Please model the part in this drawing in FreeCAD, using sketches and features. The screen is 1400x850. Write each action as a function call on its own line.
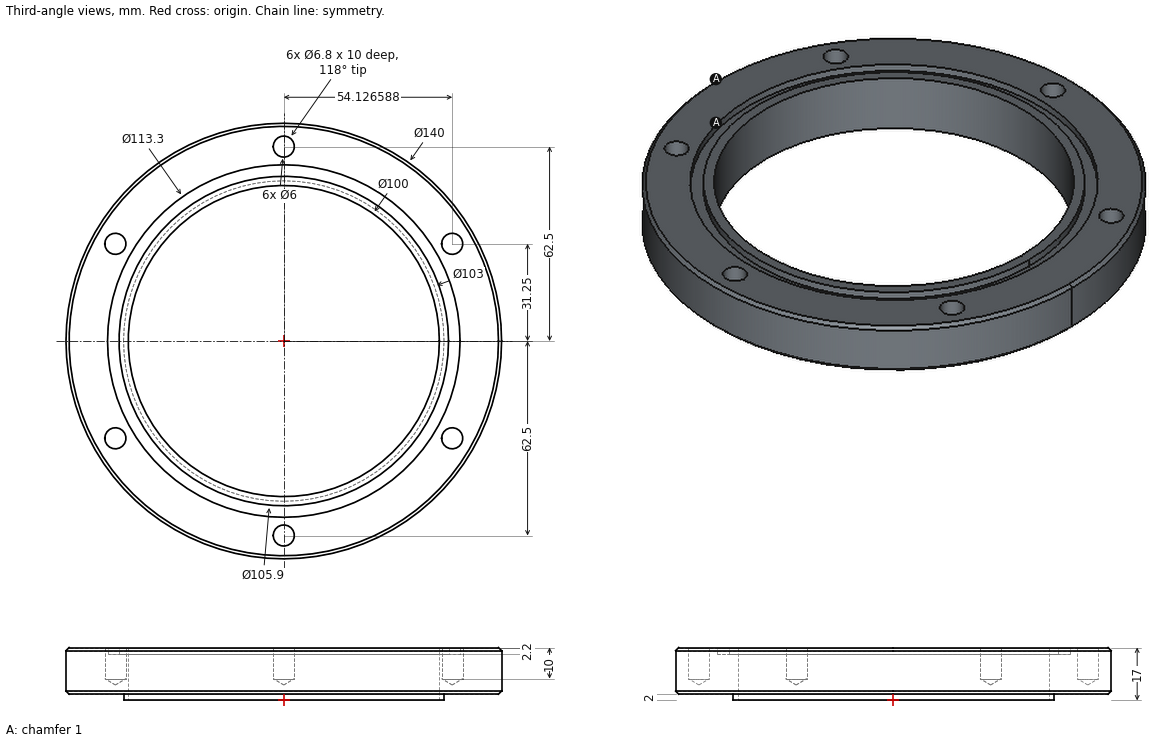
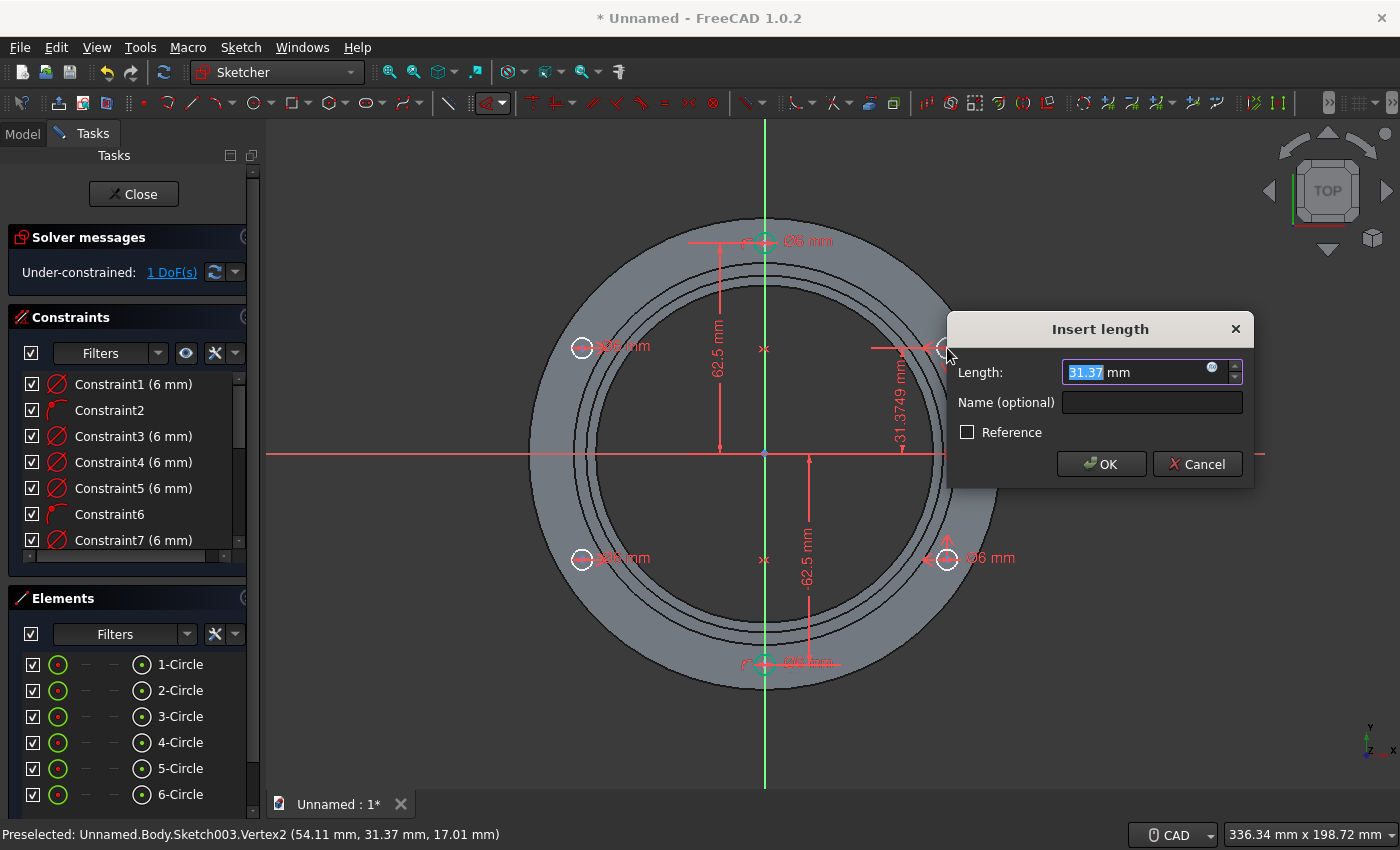
text(31.25)
key(Return)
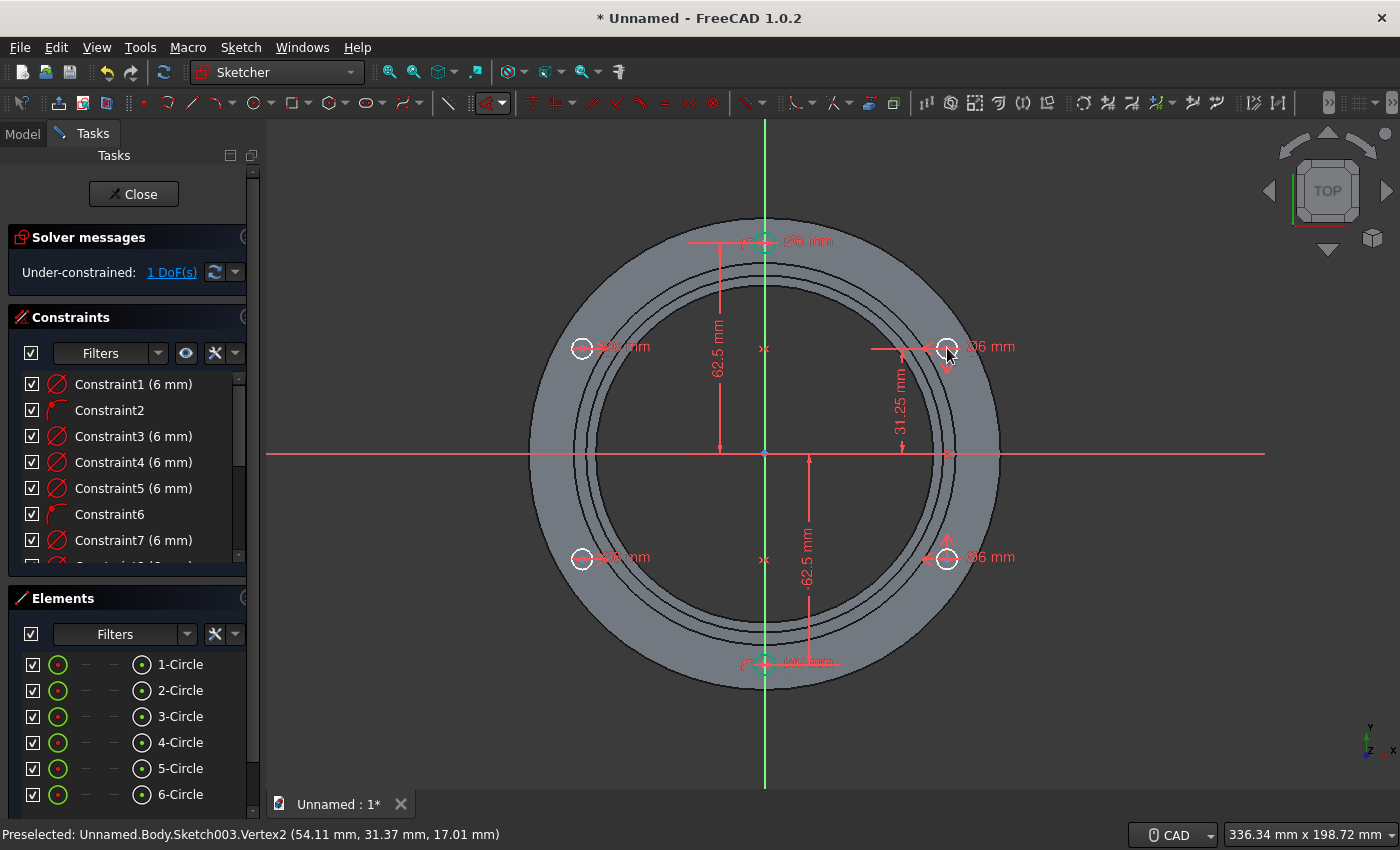
click(947, 349)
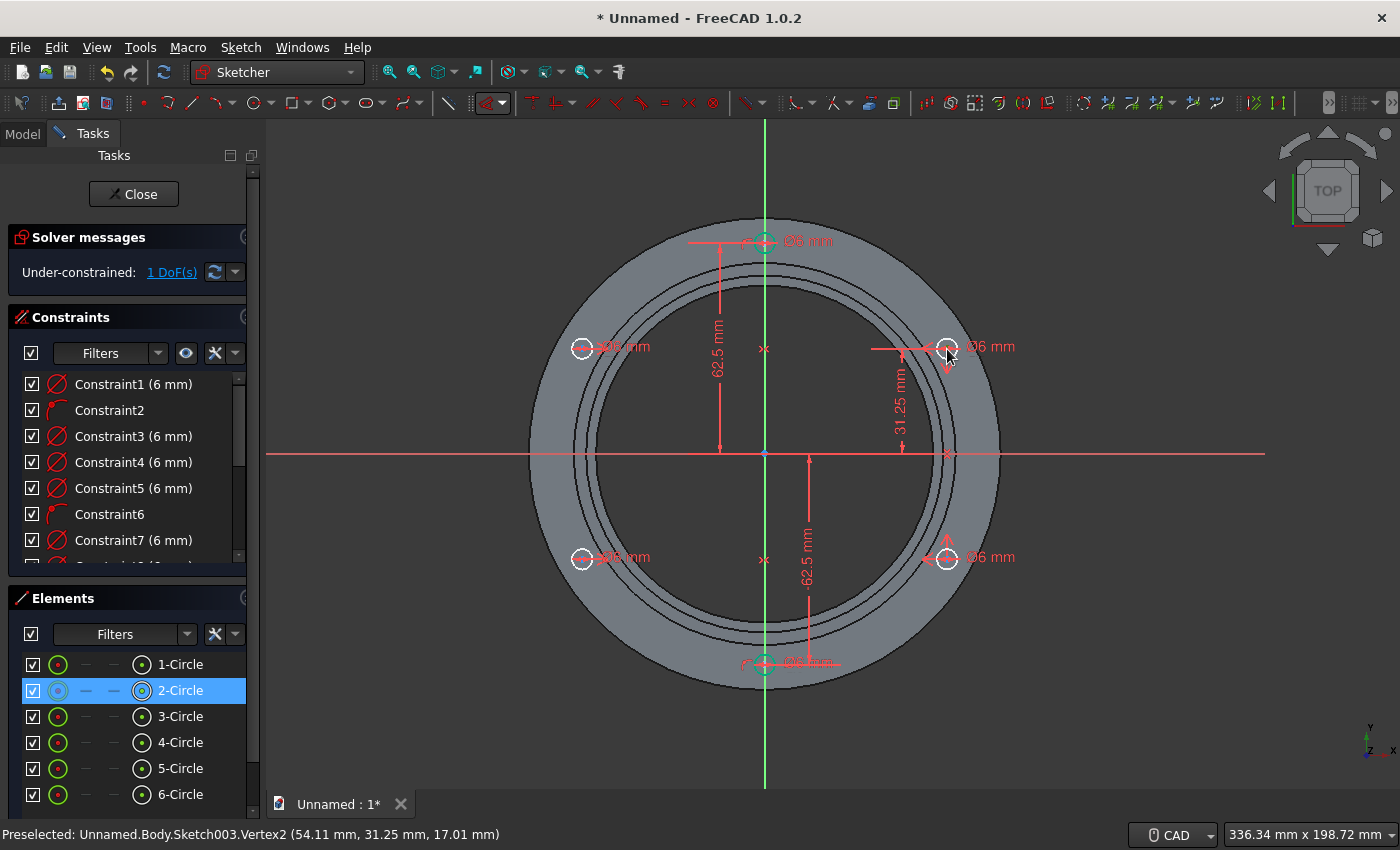
click(504, 104)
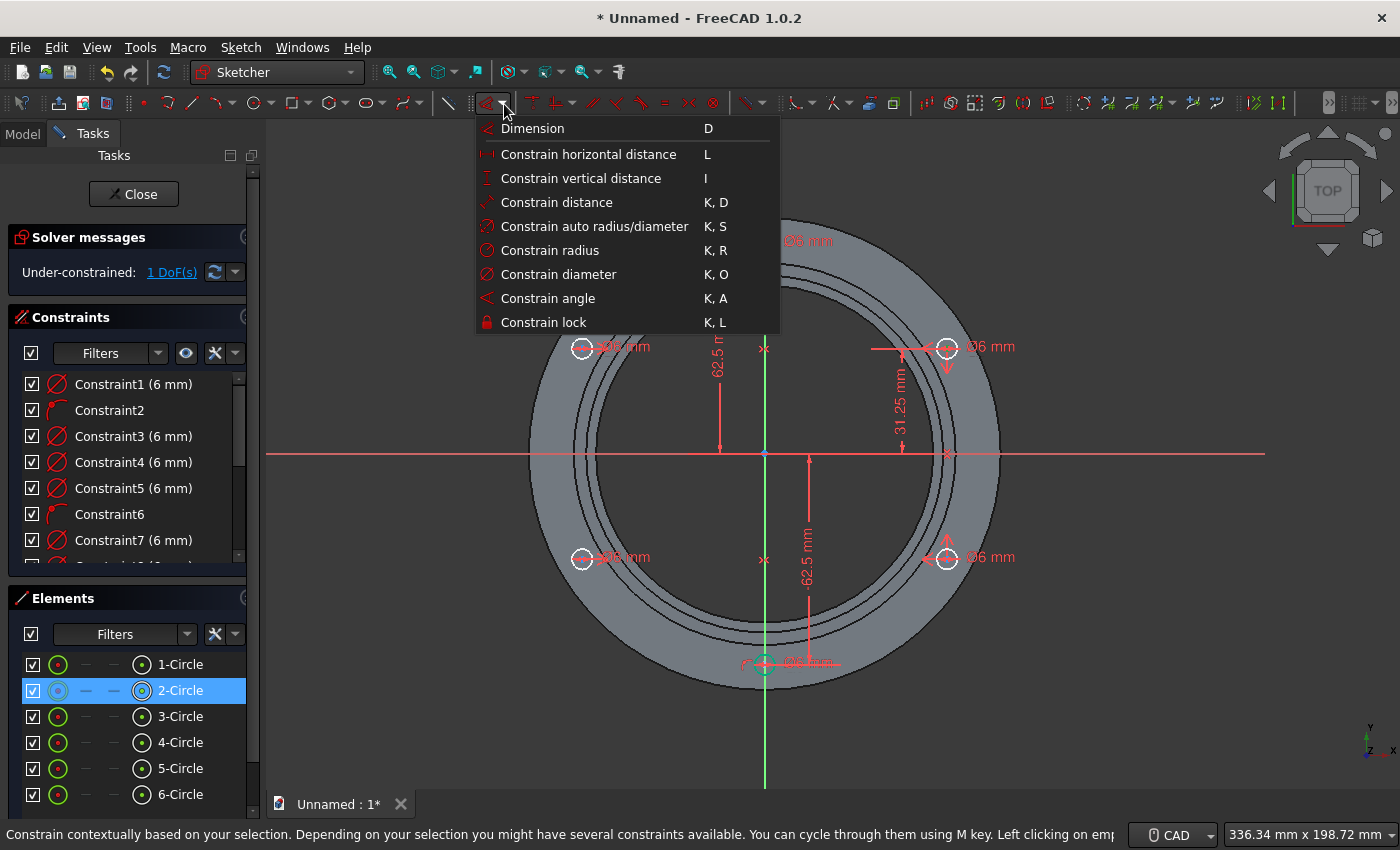
click(628, 154)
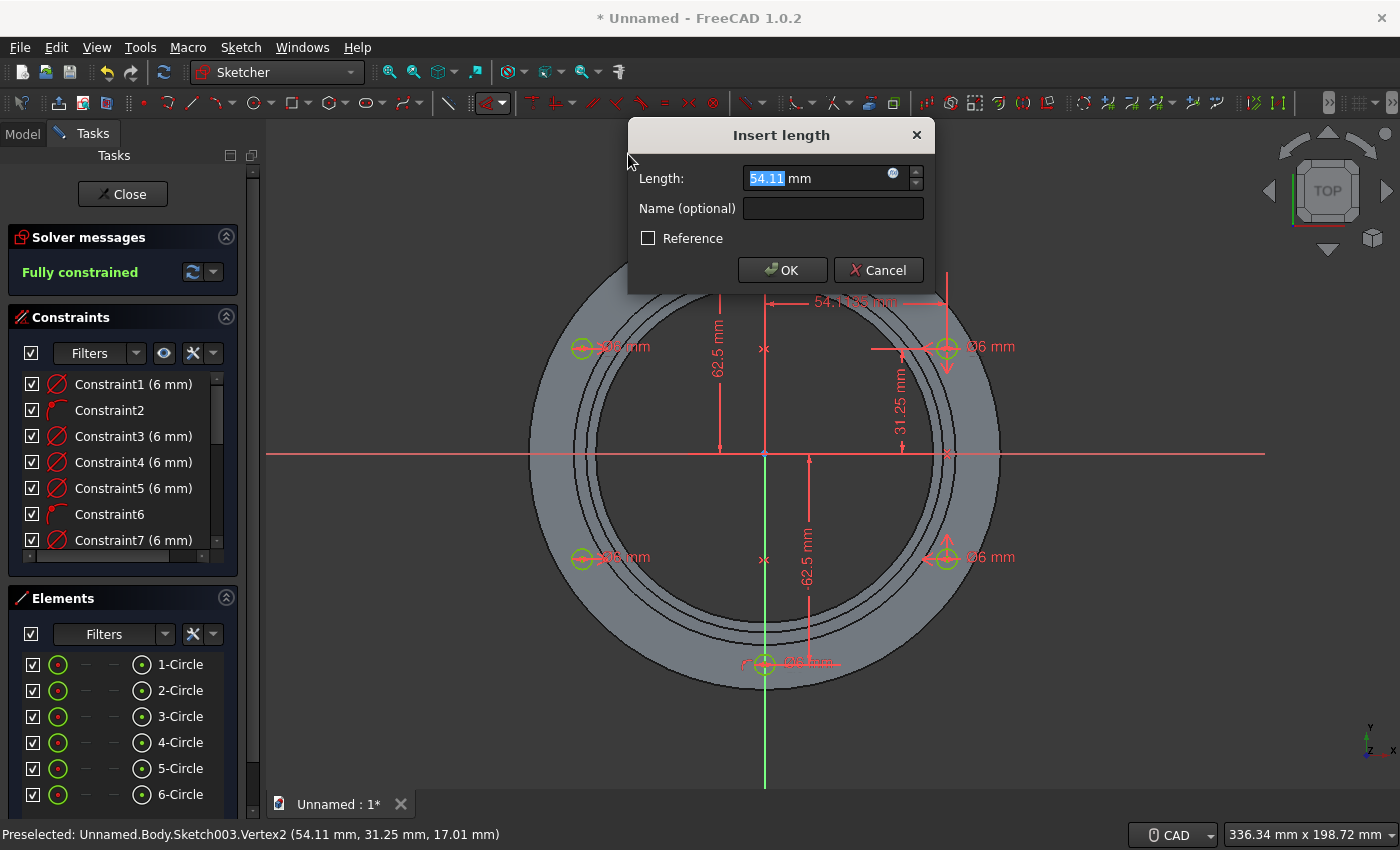
text(54.126588)
key(Return)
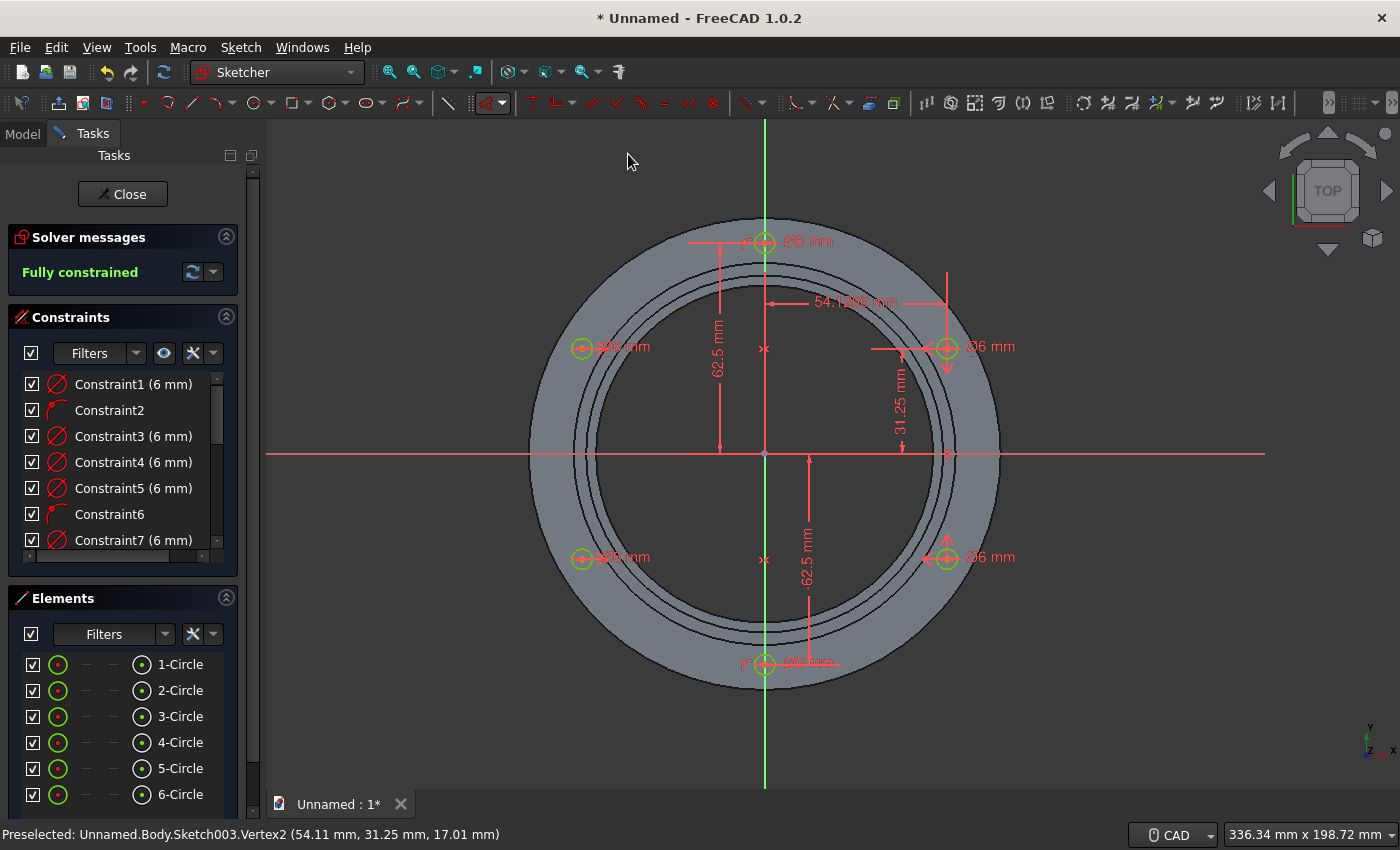
click(123, 194)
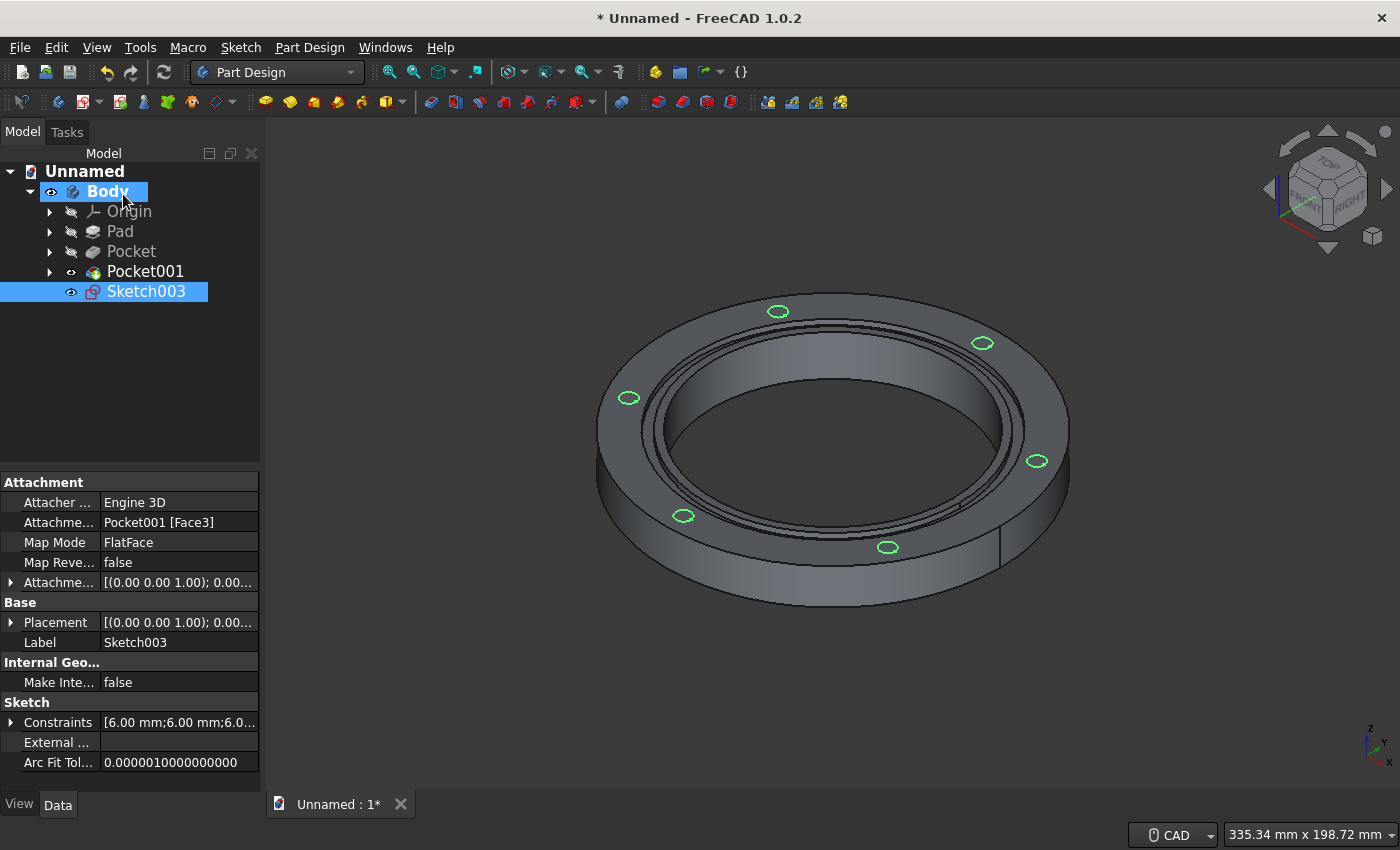
click(432, 102)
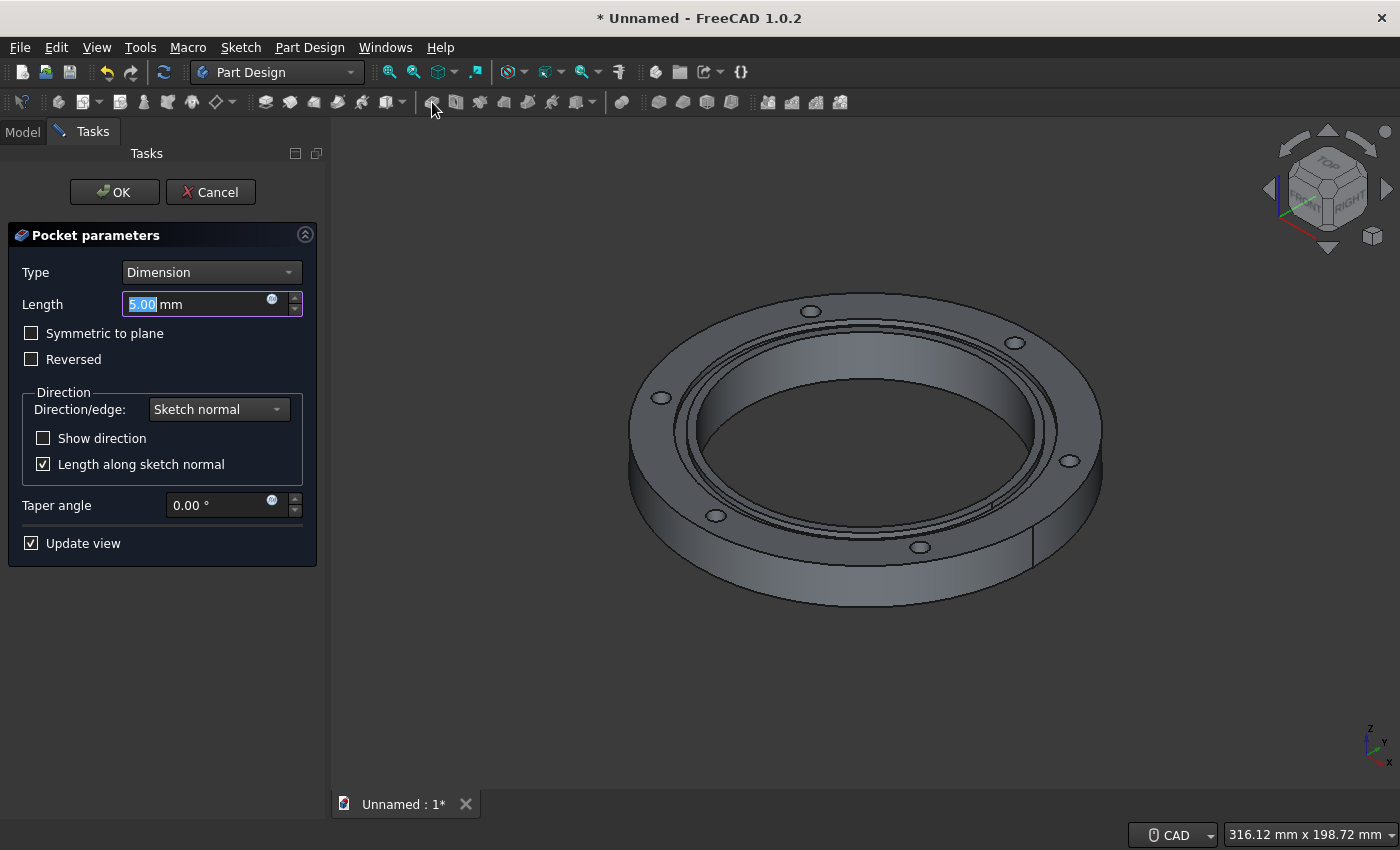
text(10)
key(Tab)